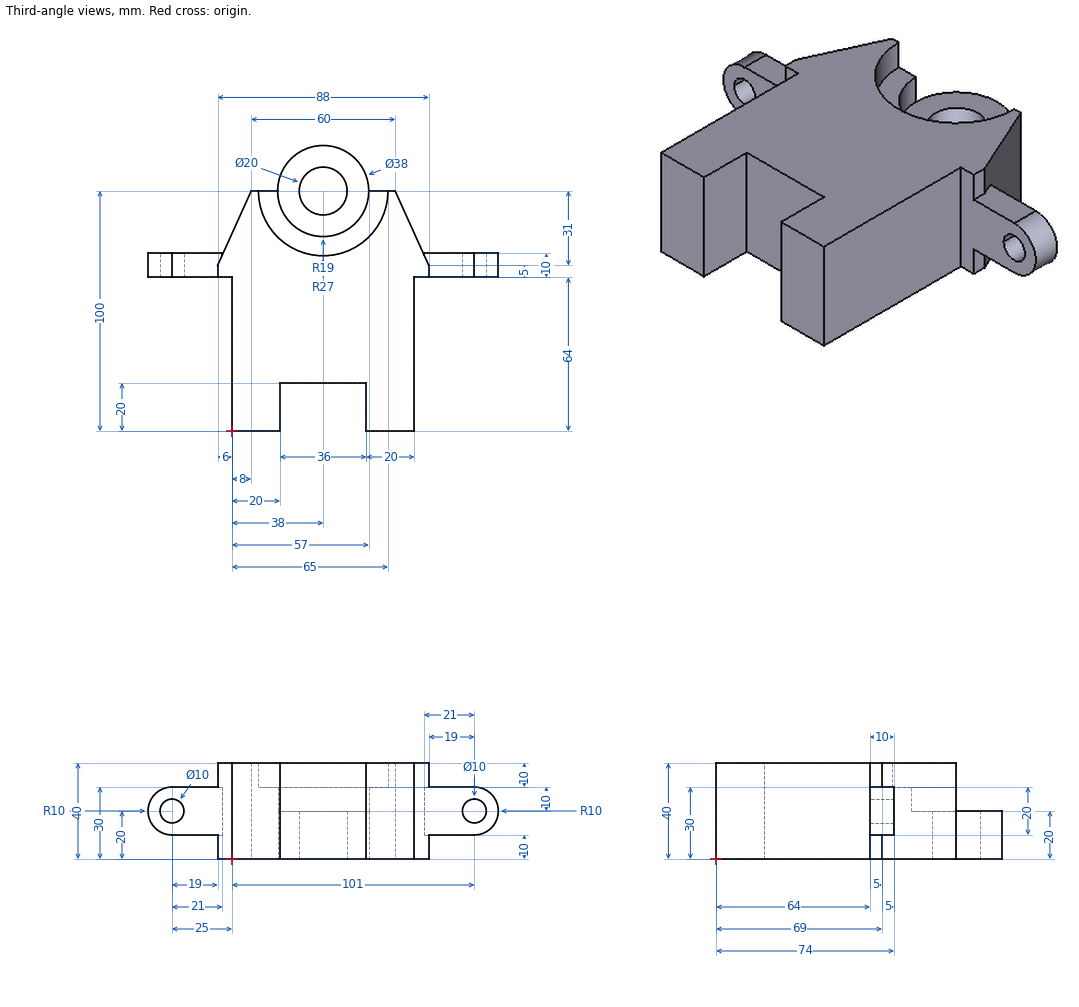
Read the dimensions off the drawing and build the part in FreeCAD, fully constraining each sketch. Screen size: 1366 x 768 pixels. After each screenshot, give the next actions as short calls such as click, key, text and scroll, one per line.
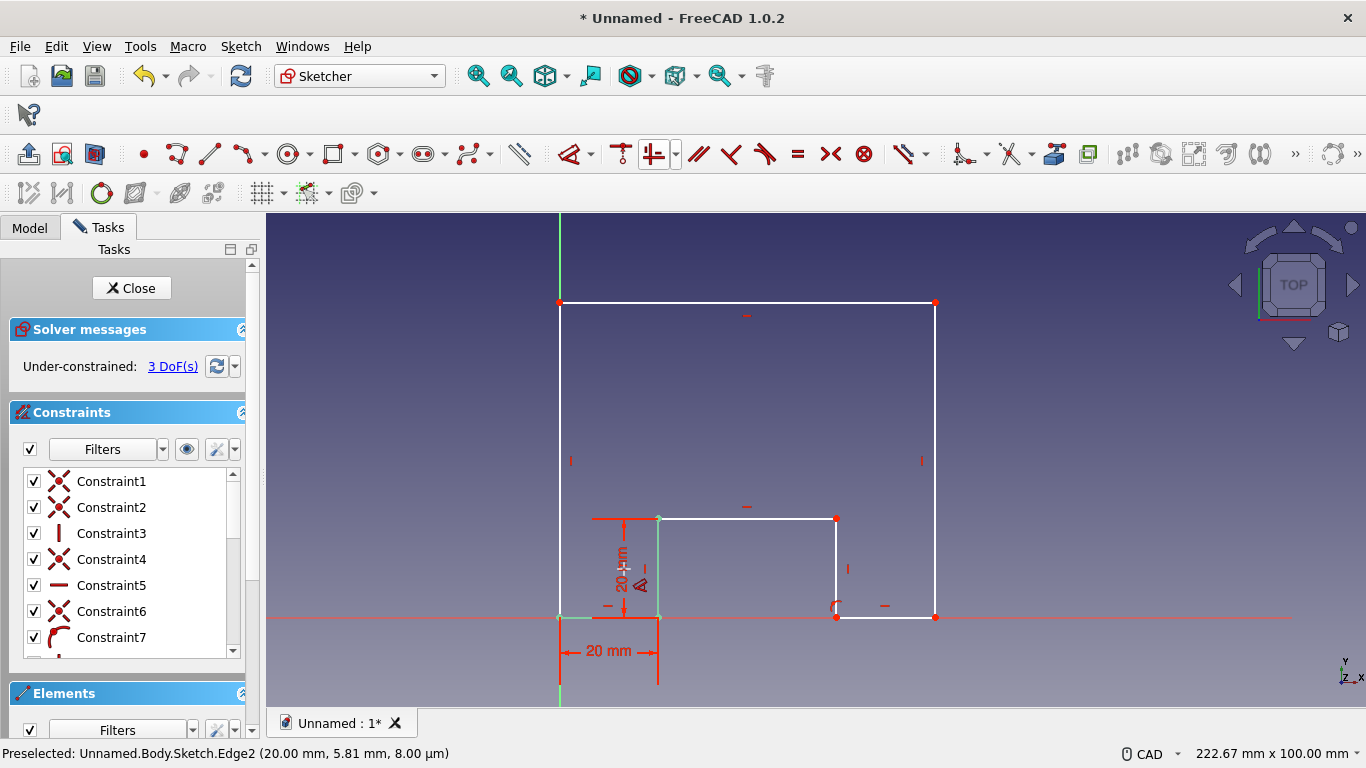
click(712, 519)
click(747, 553)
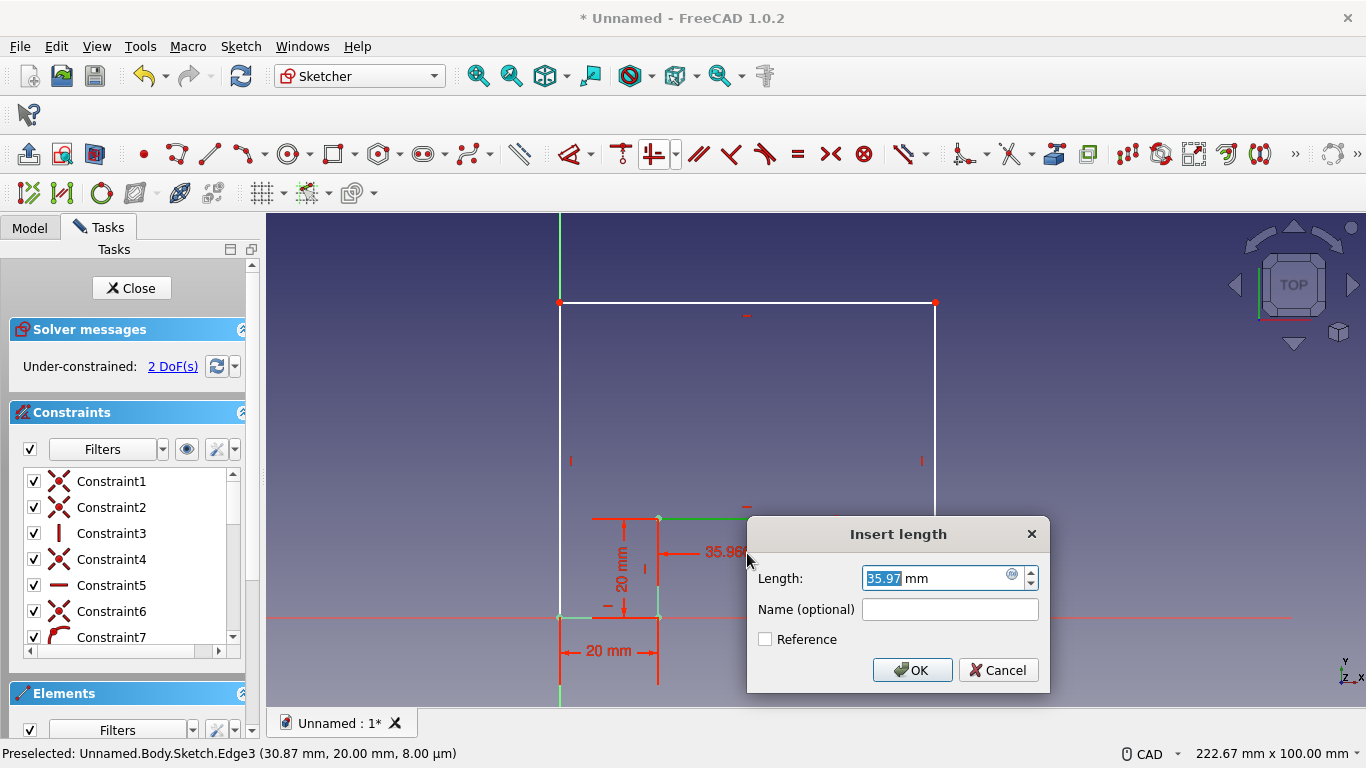
text(36)
key(Return)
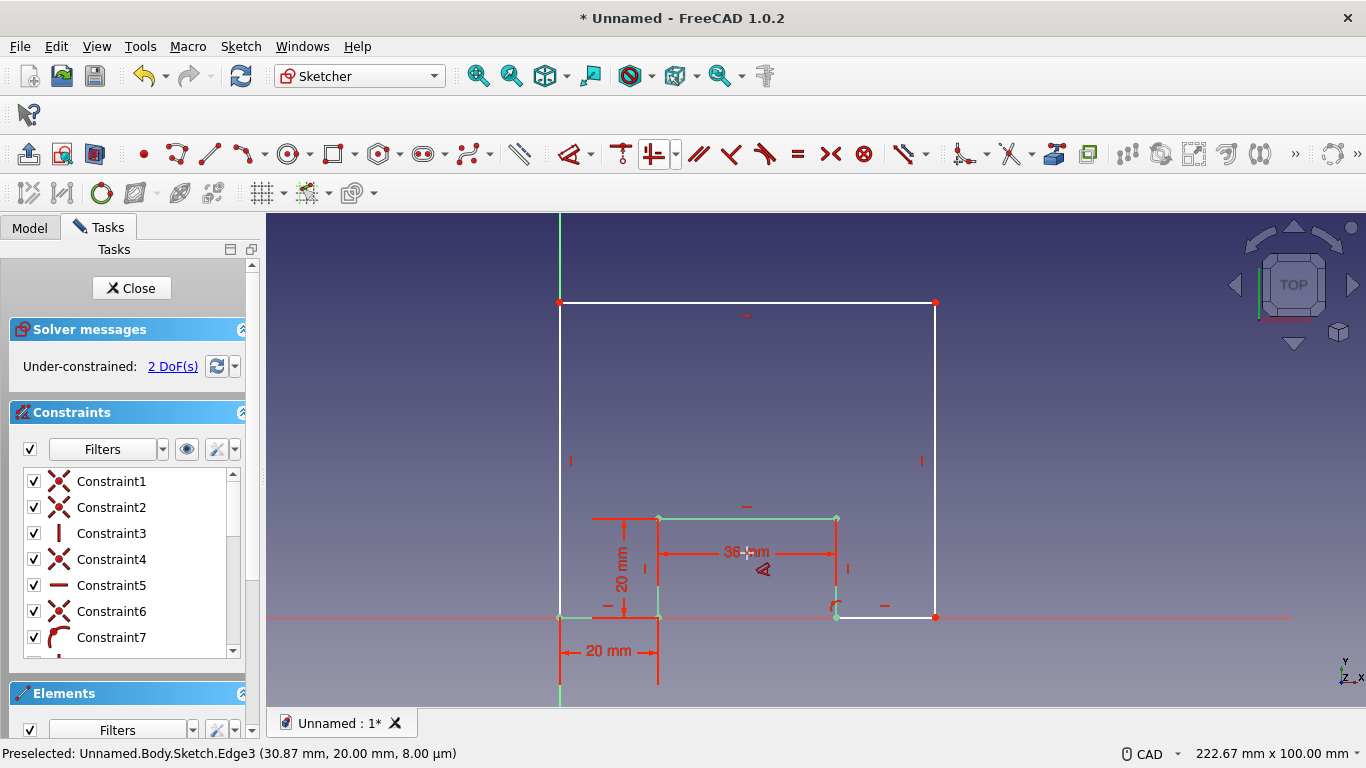
click(866, 618)
click(886, 652)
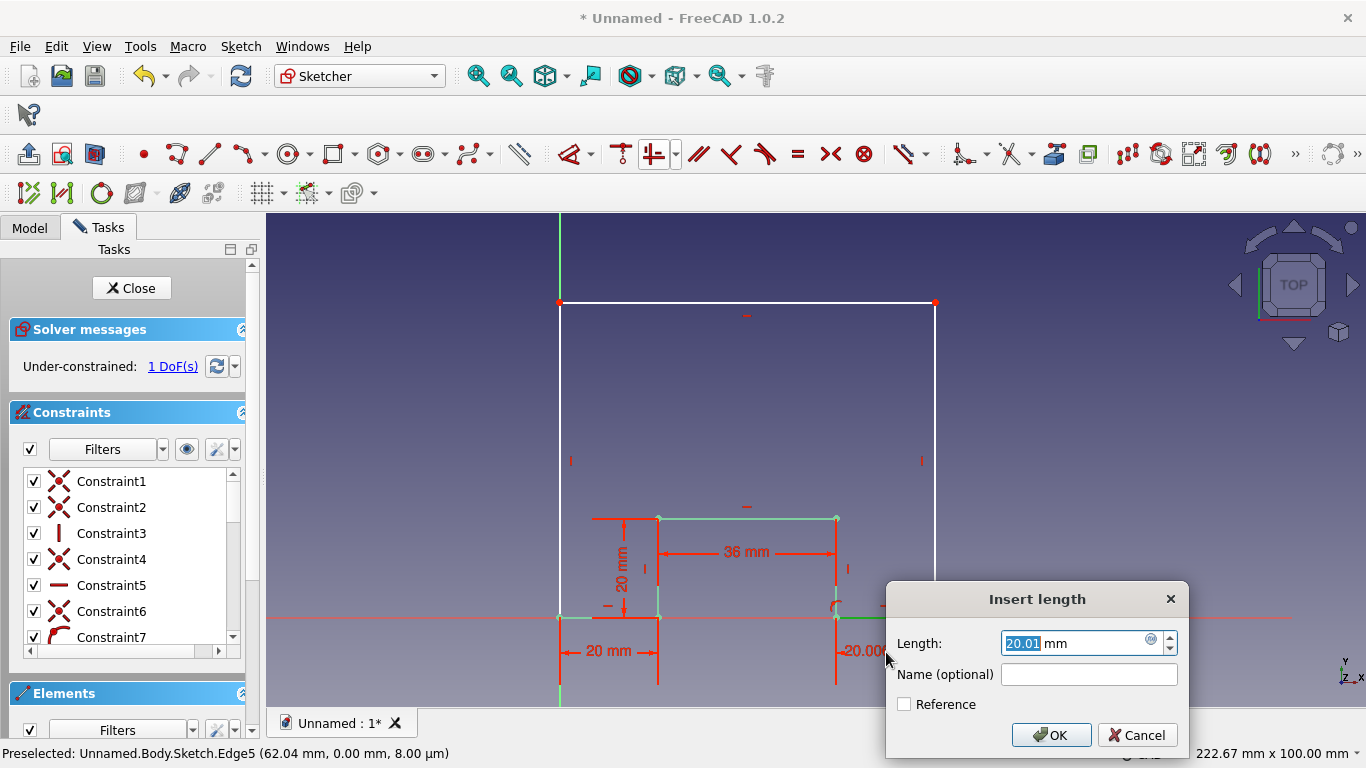
text(20)
key(Return)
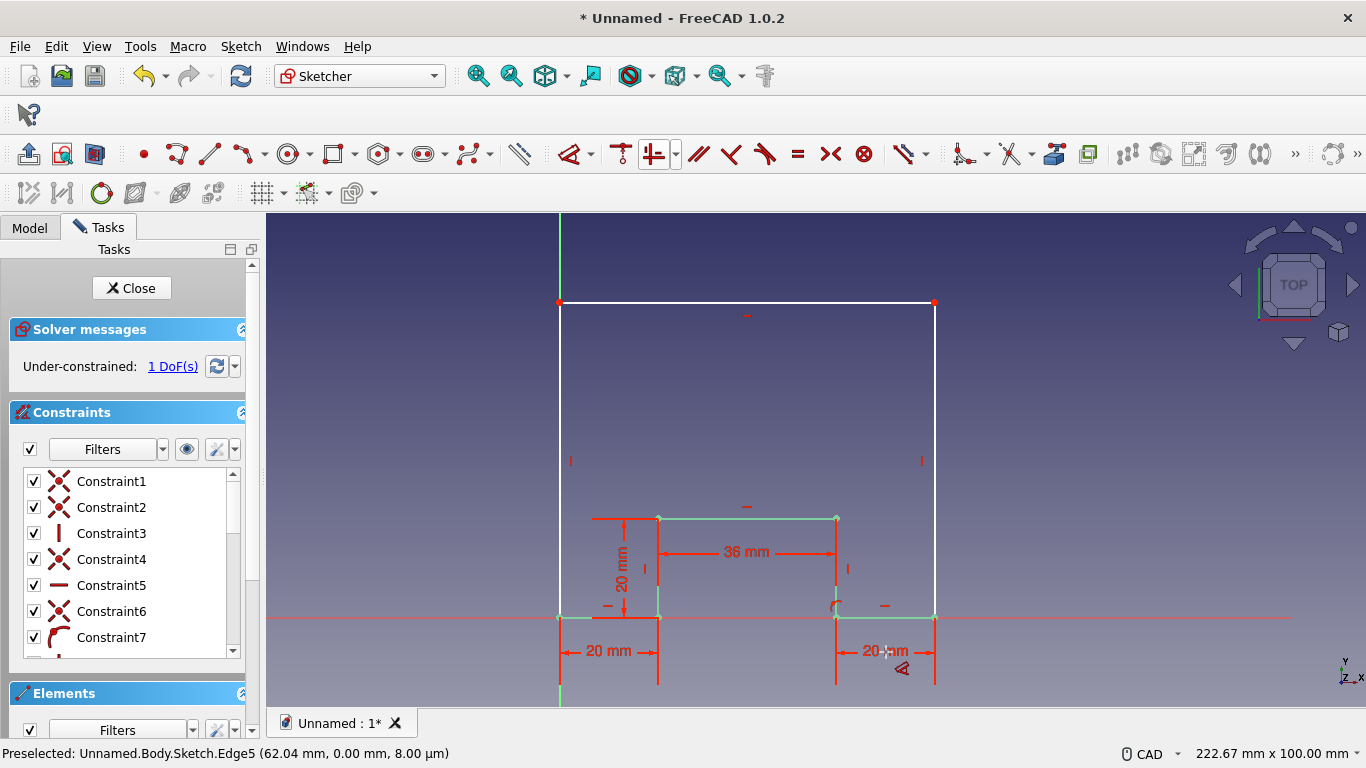
click(935, 523)
click(969, 460)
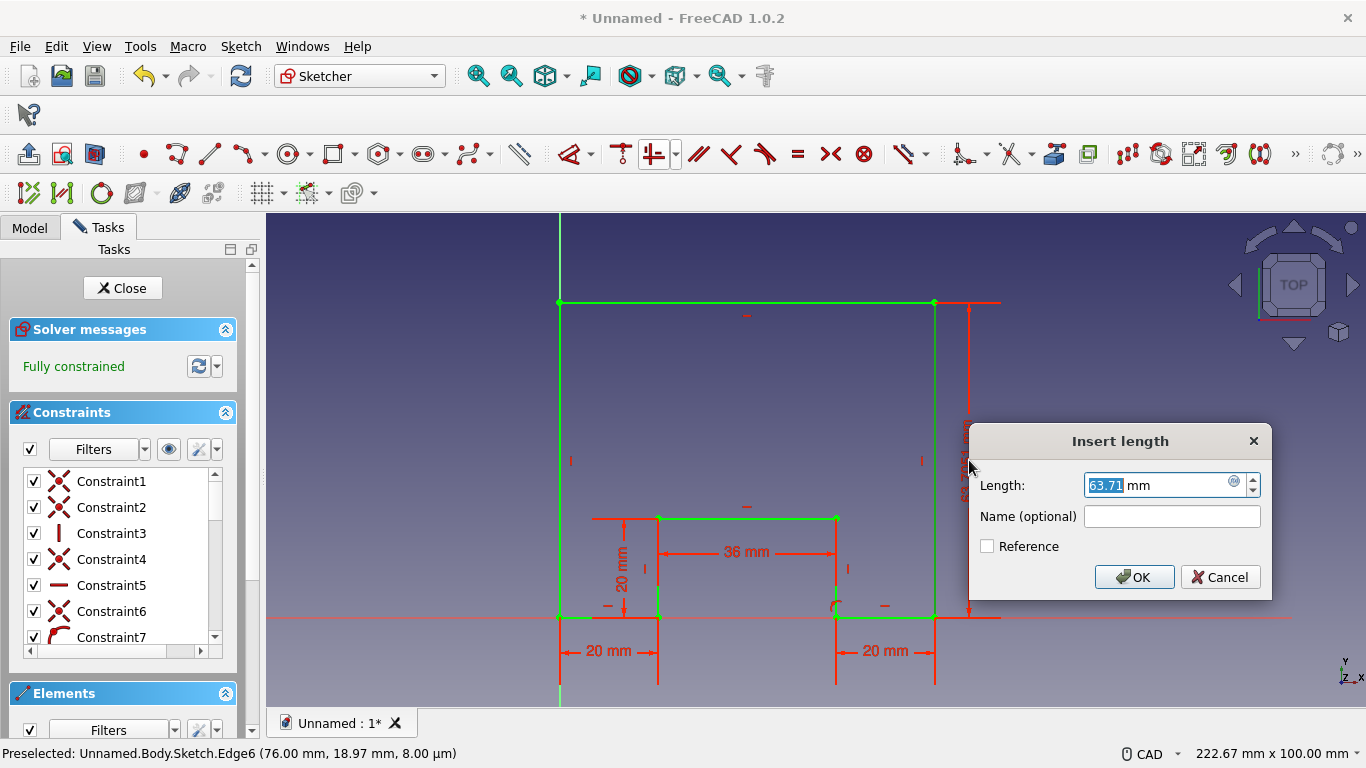
text(64)
key(Return)
key(Escape)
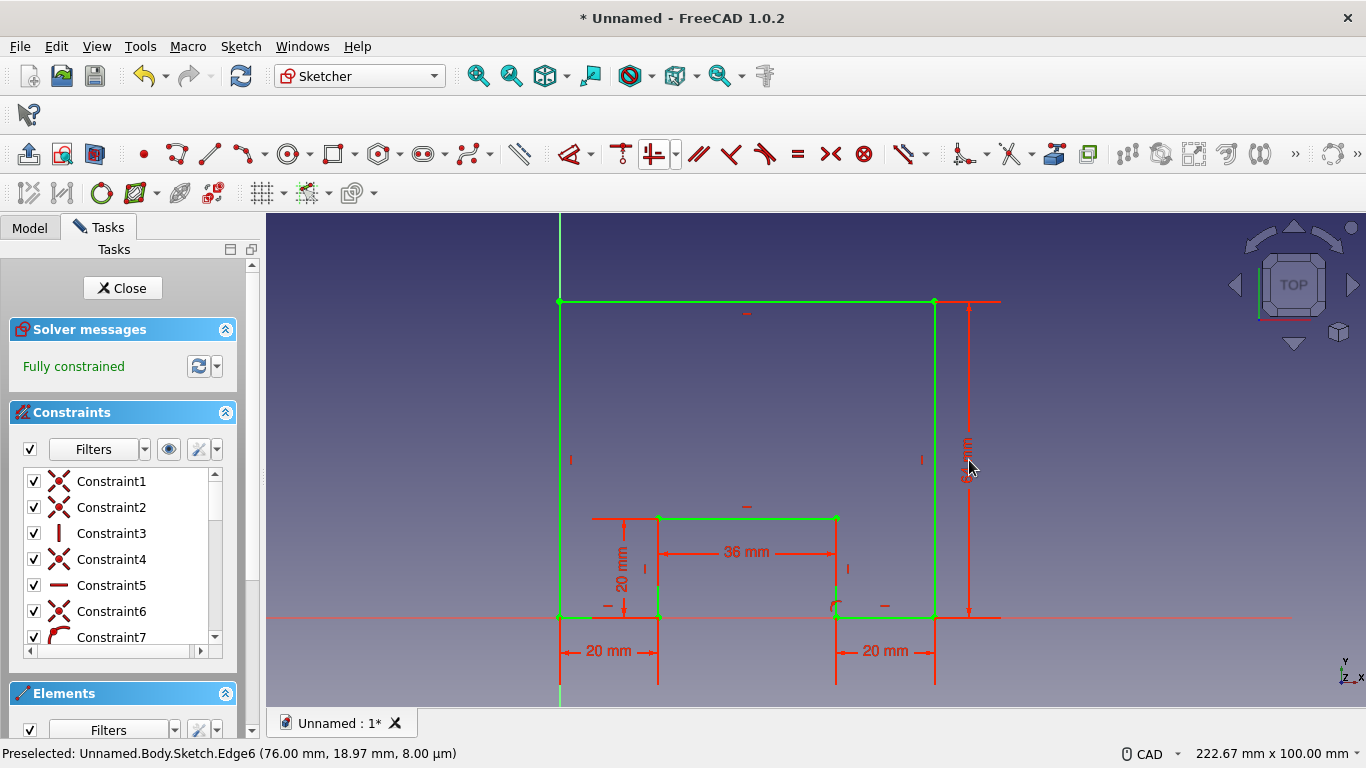
click(123, 288)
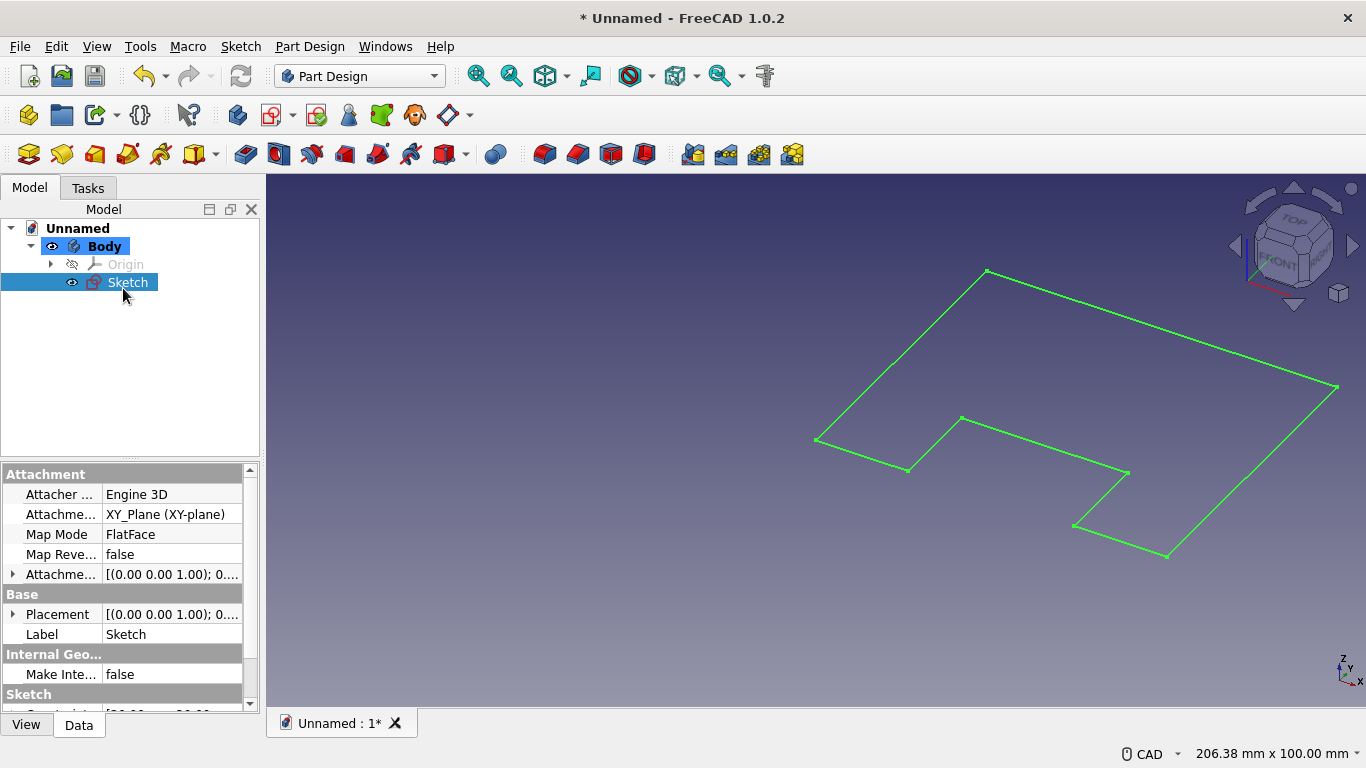
click(29, 154)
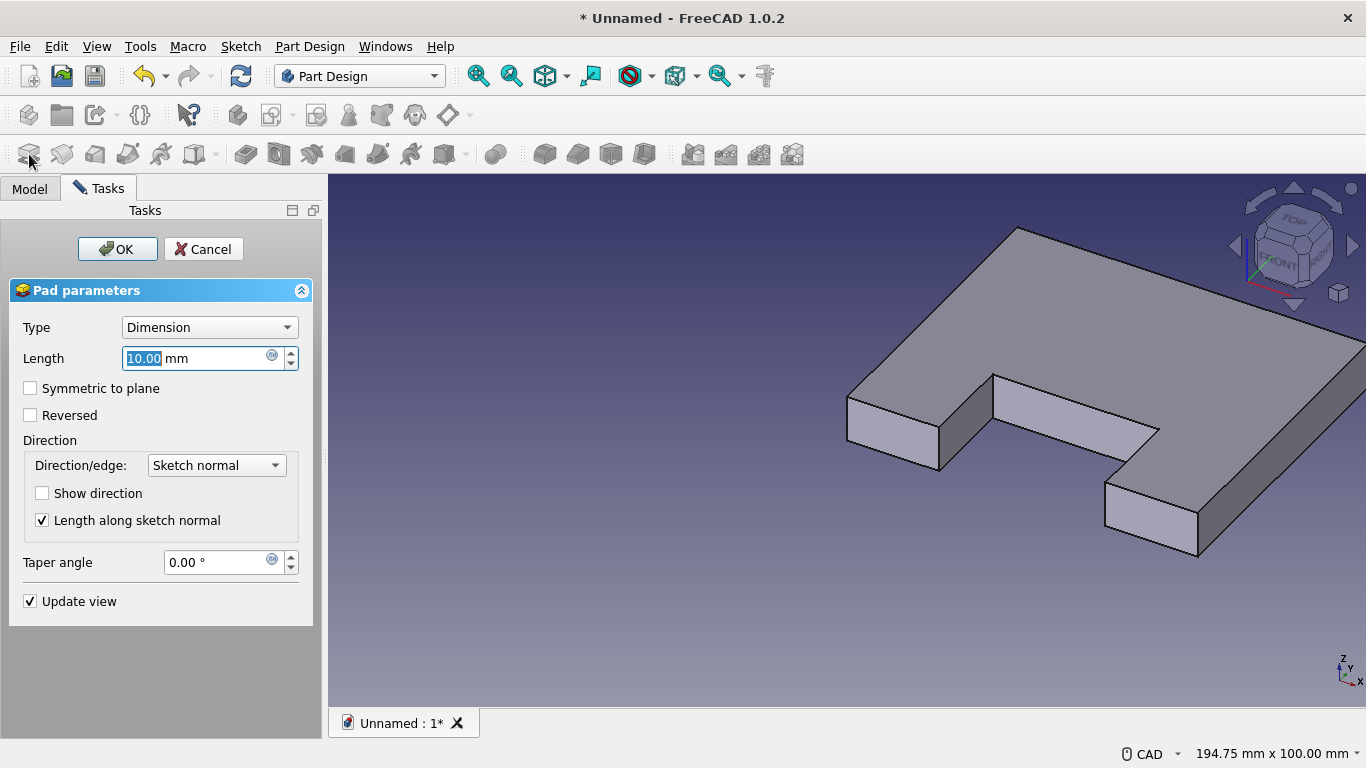
text(40)
key(Tab)